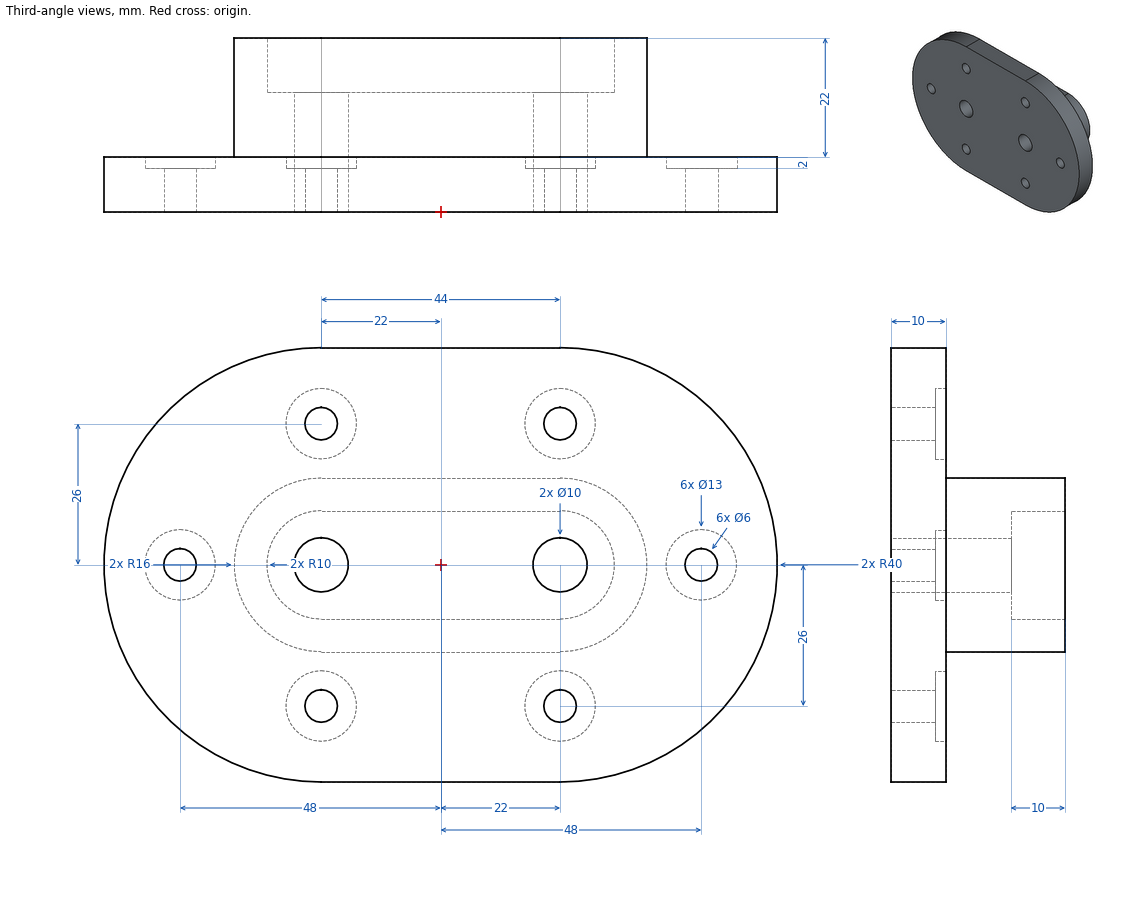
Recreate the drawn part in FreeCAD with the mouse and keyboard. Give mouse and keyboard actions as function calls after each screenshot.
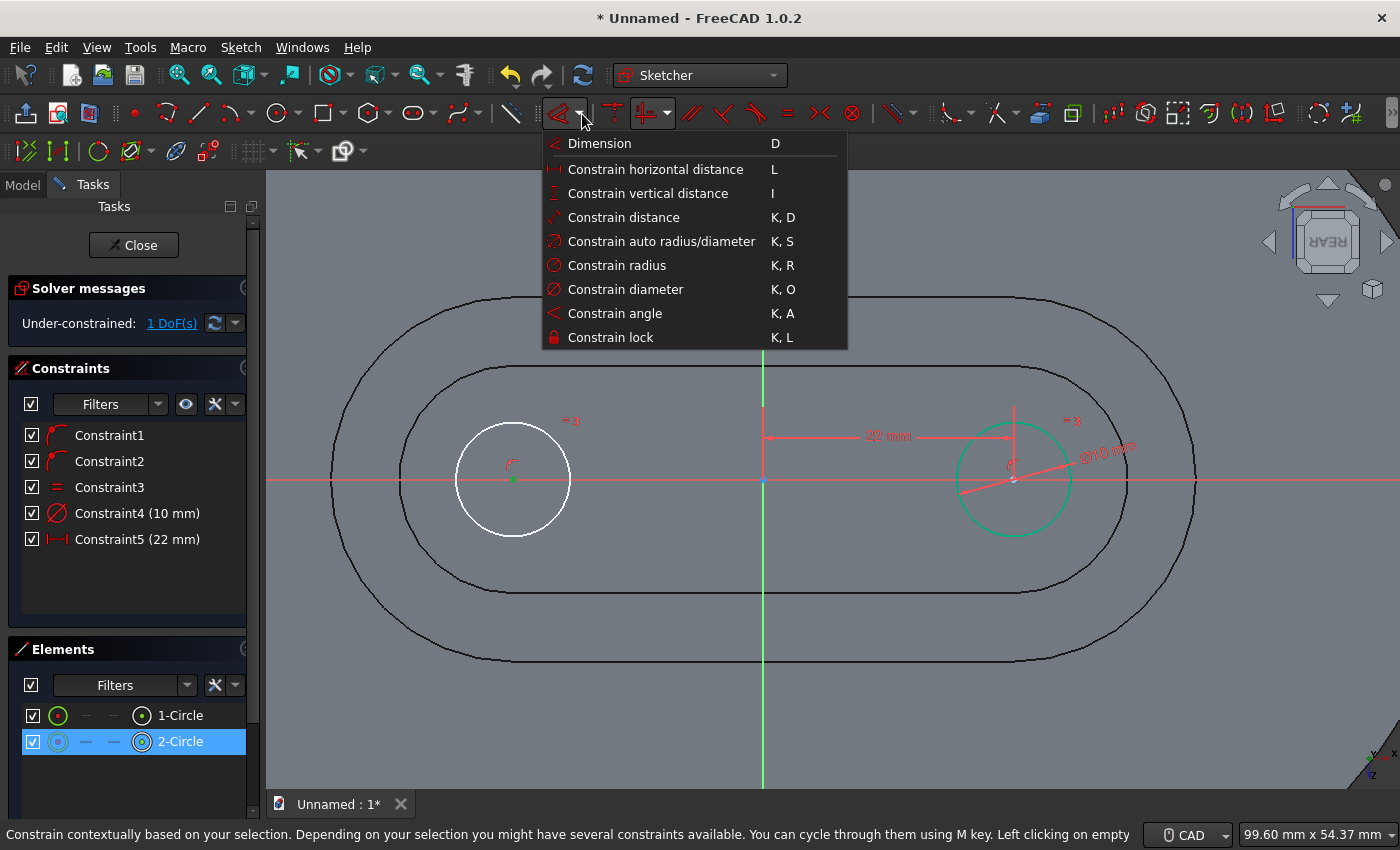
click(695, 169)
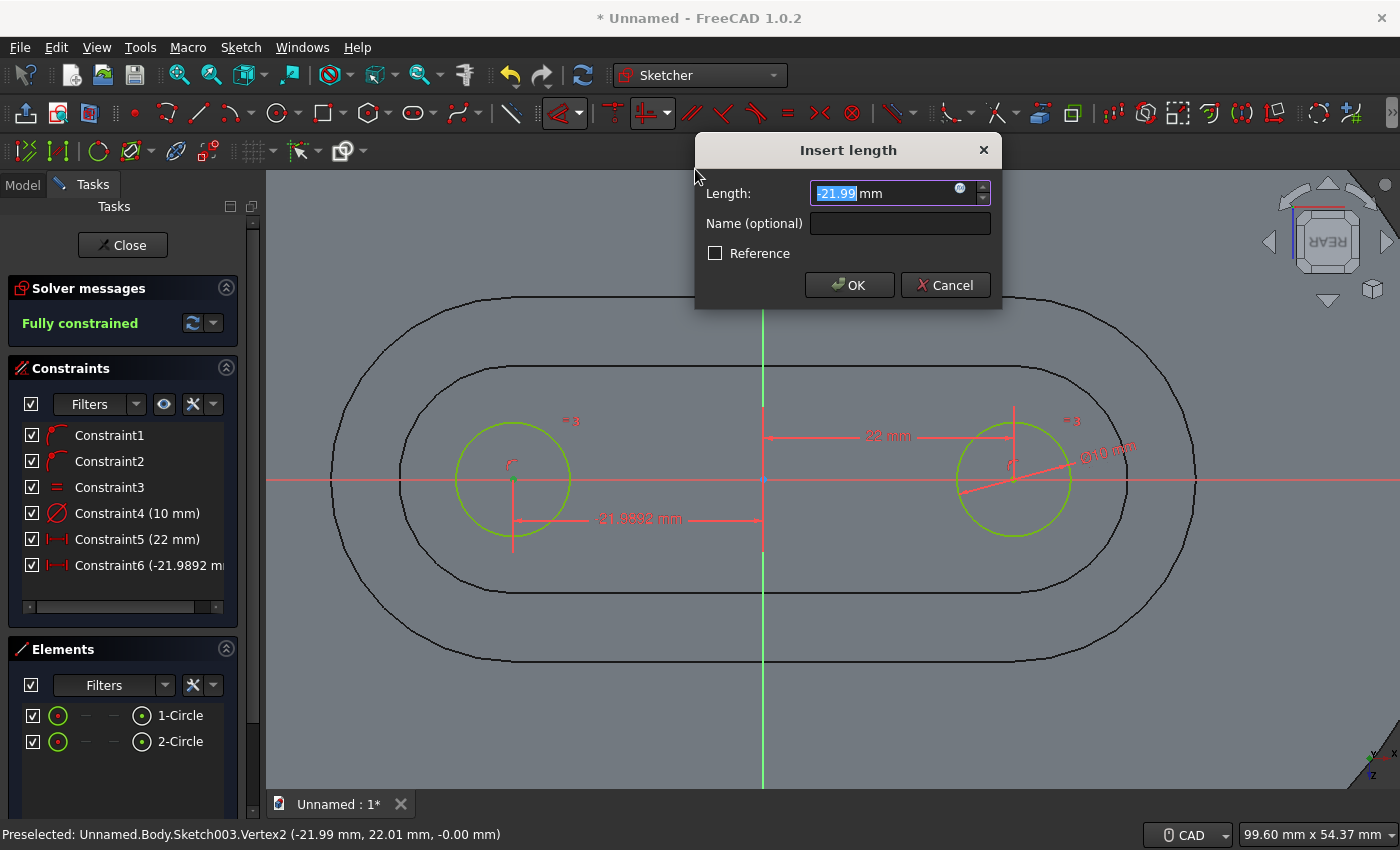
text(-22)
key(Return)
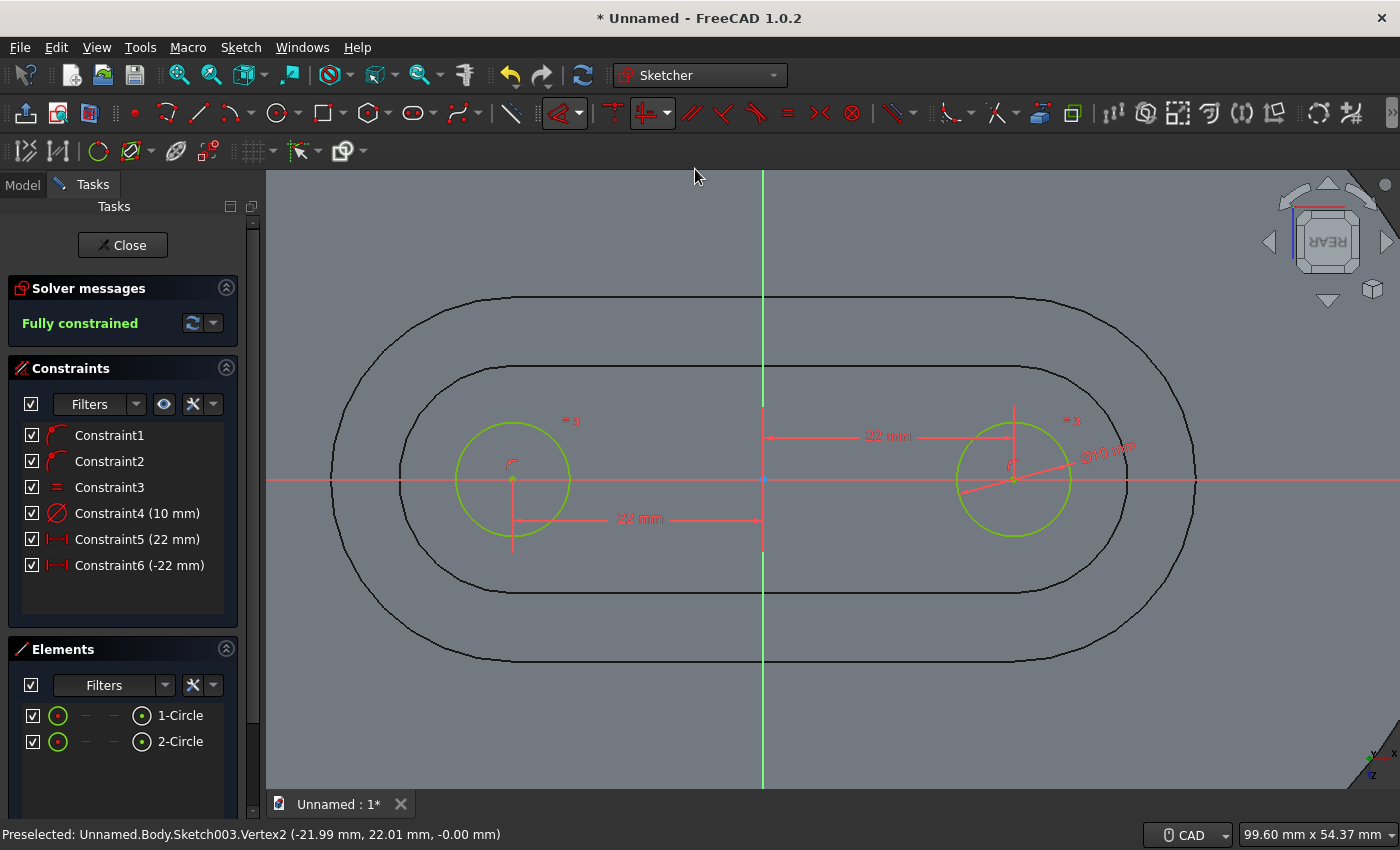
click(123, 245)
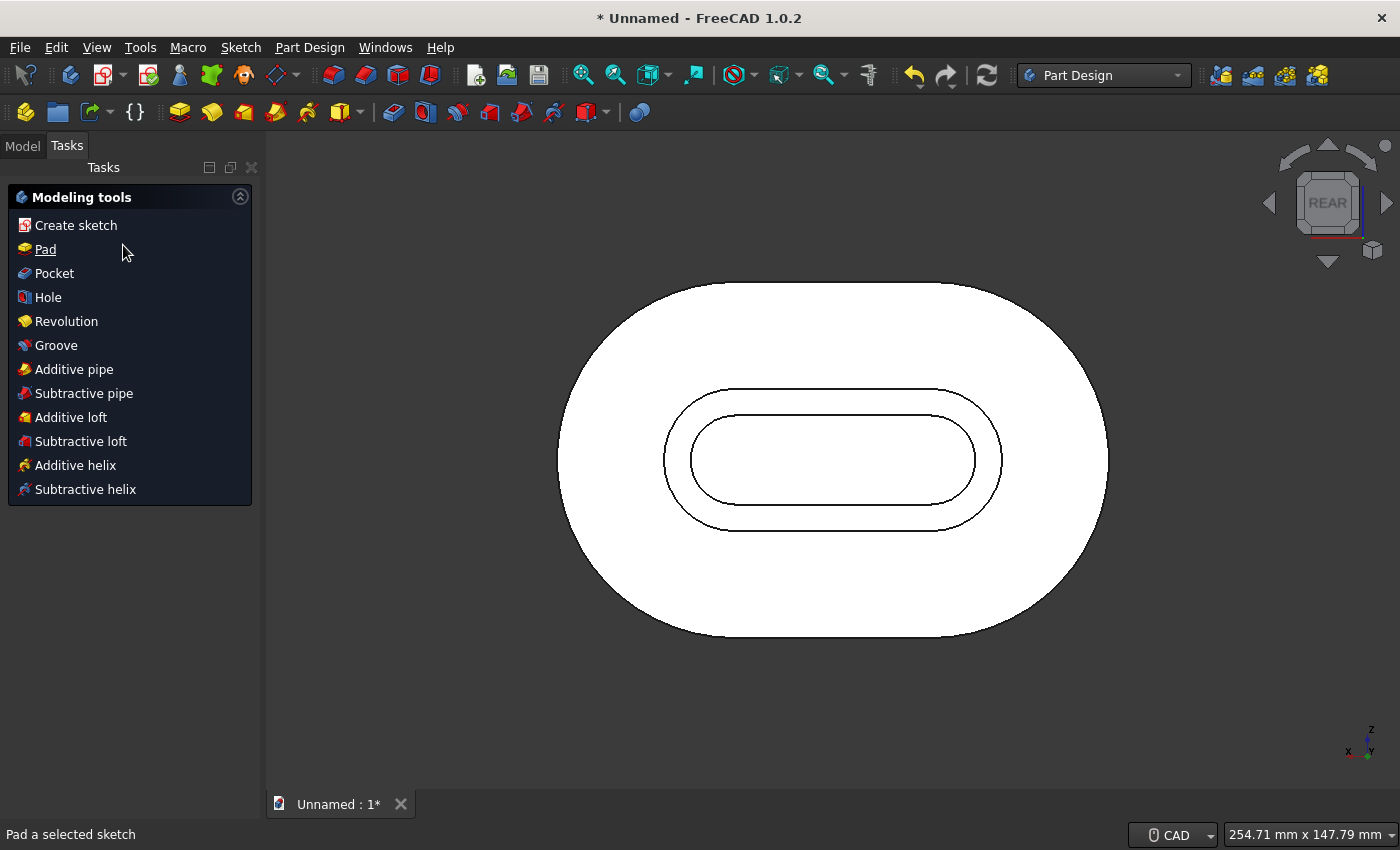
click(394, 112)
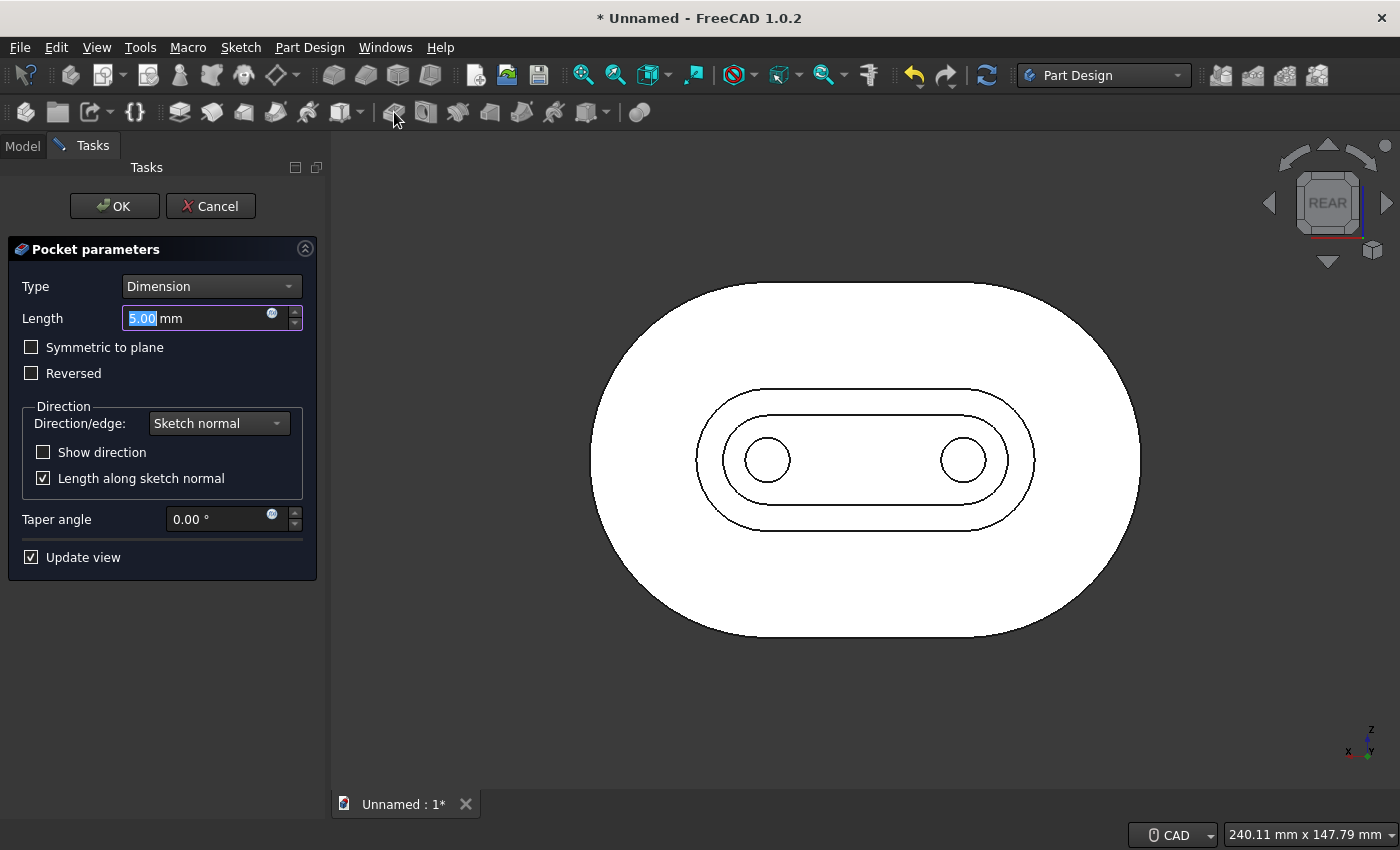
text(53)
key(Tab)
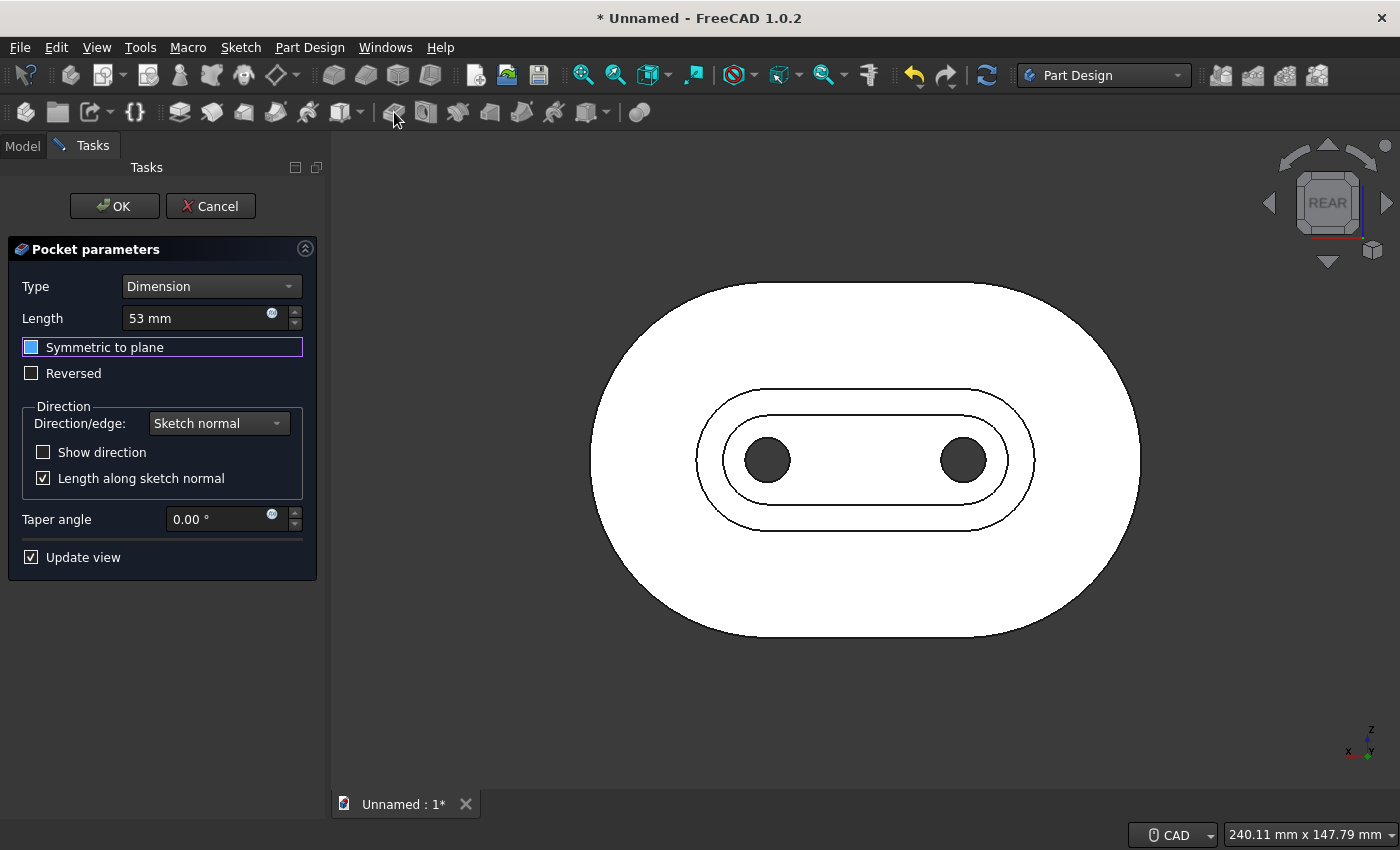
click(115, 206)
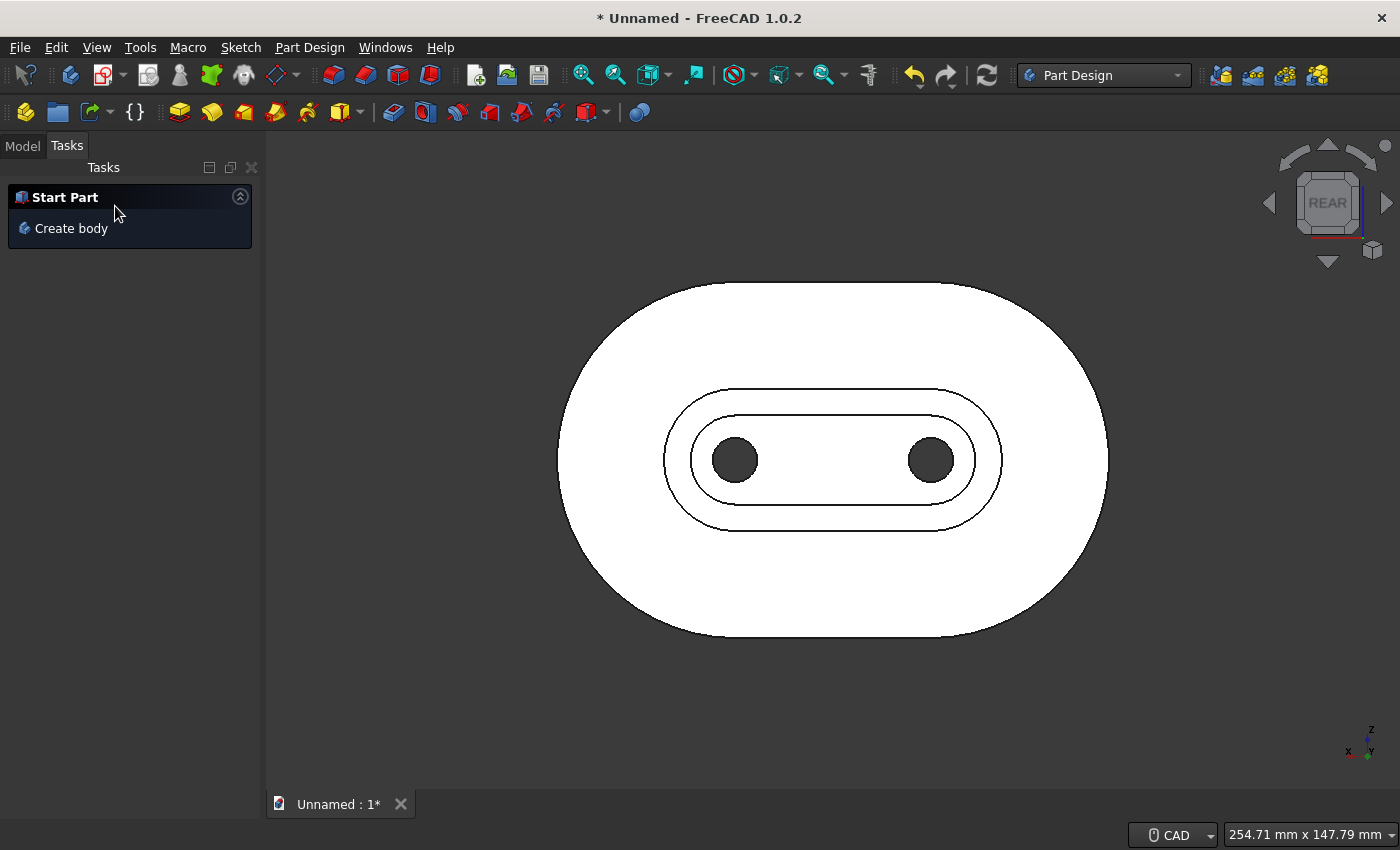
click(991, 561)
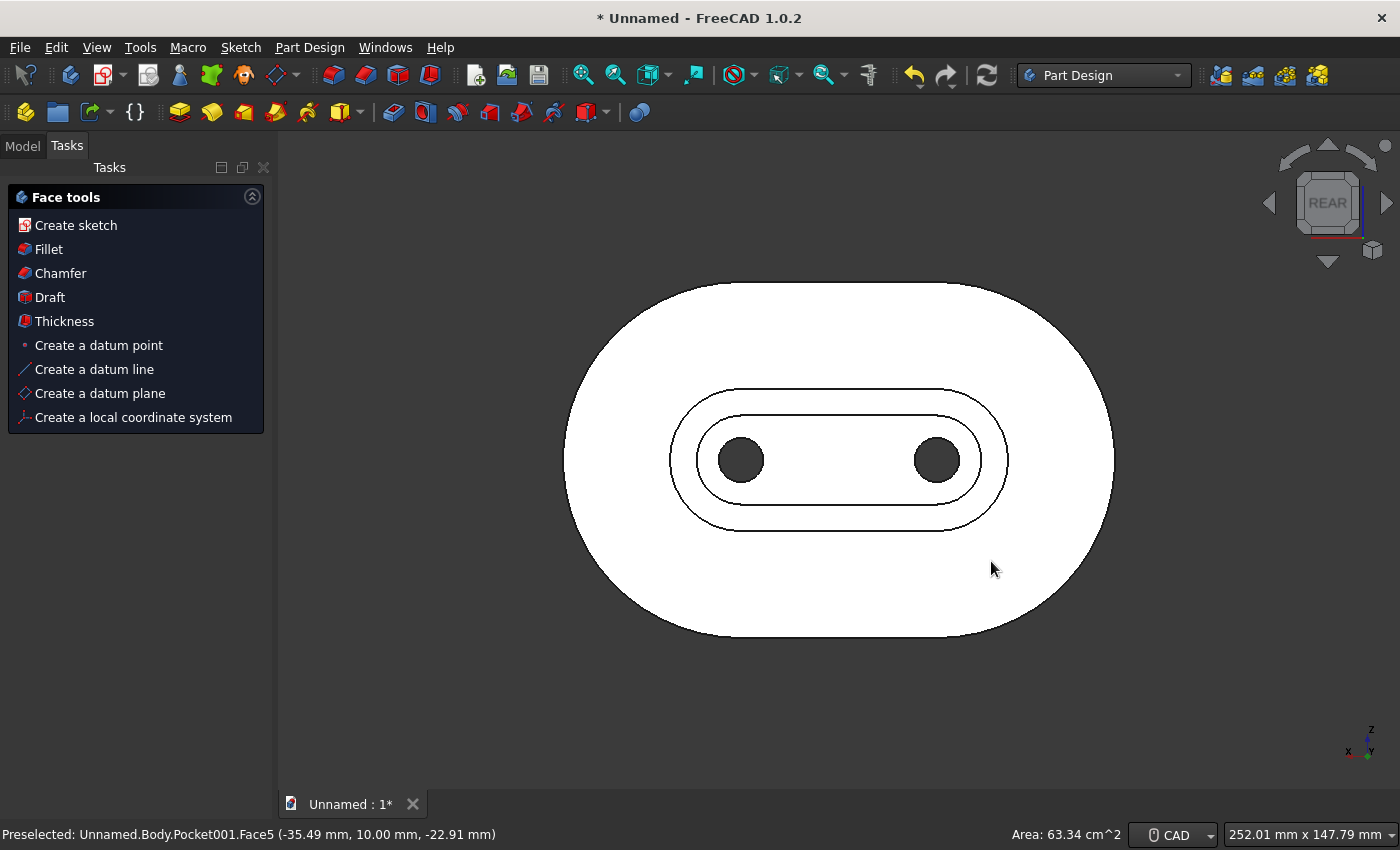
click(104, 76)